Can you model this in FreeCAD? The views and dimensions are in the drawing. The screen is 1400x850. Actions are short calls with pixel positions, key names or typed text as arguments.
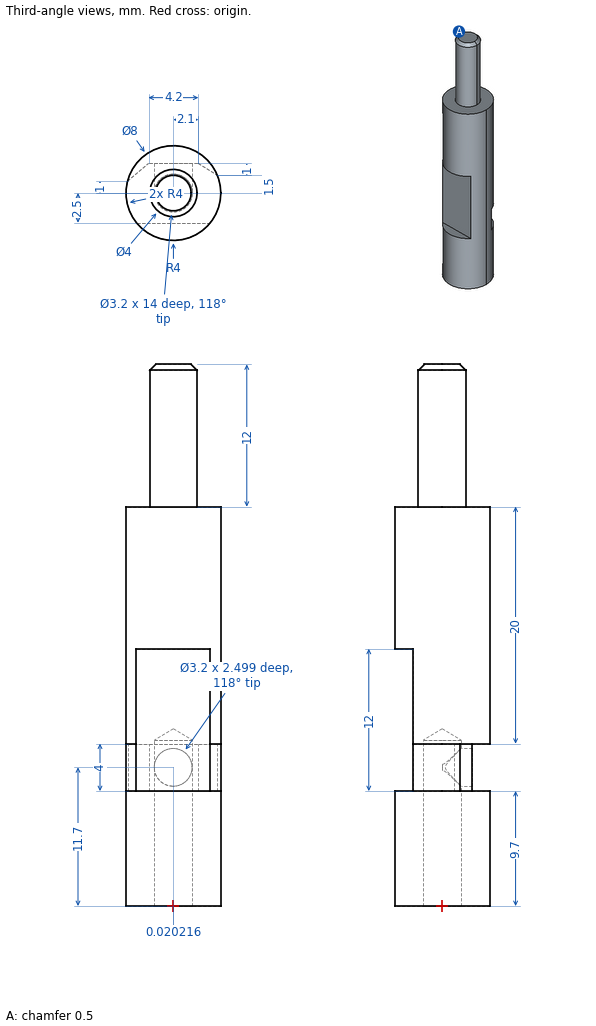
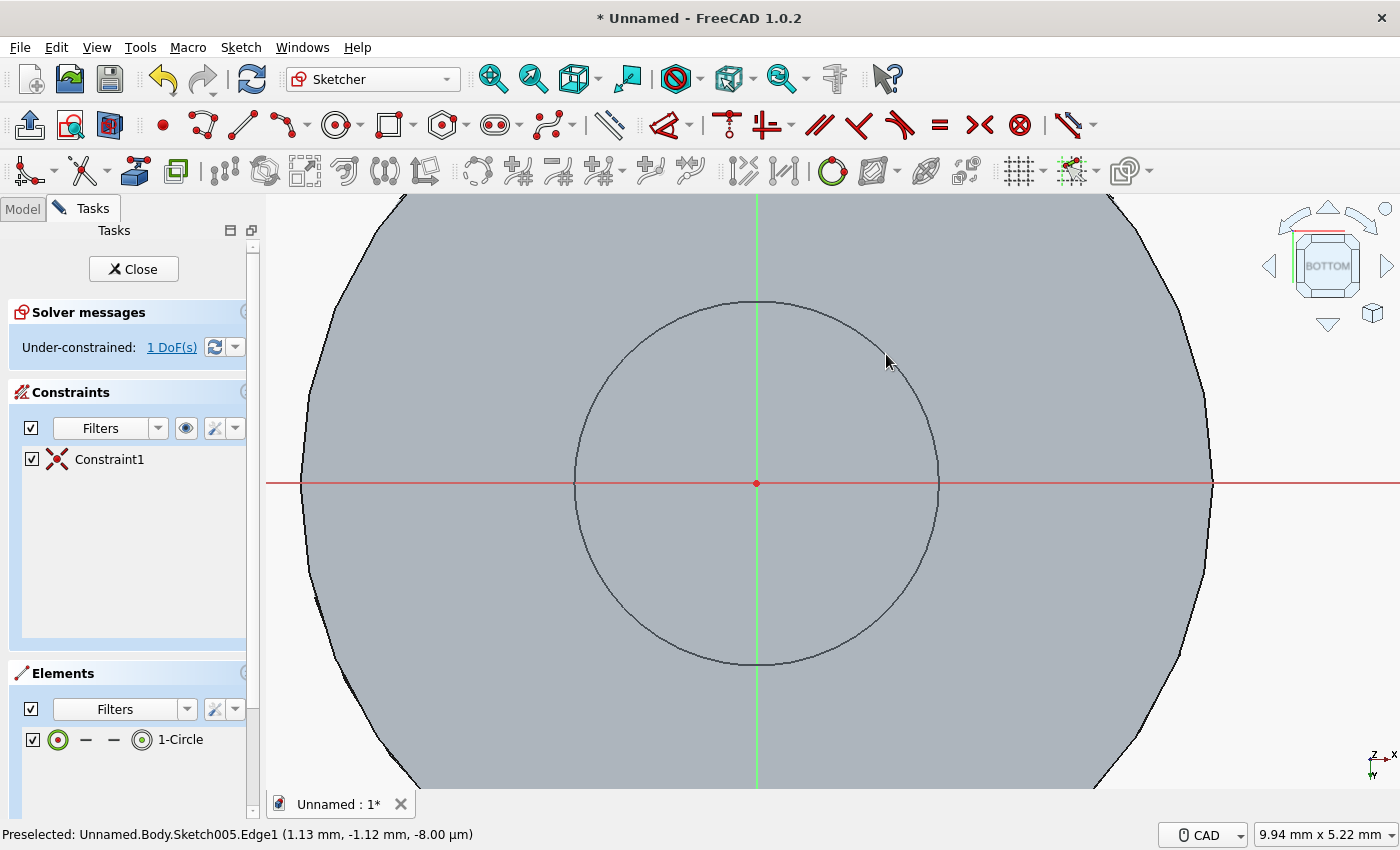
click(664, 126)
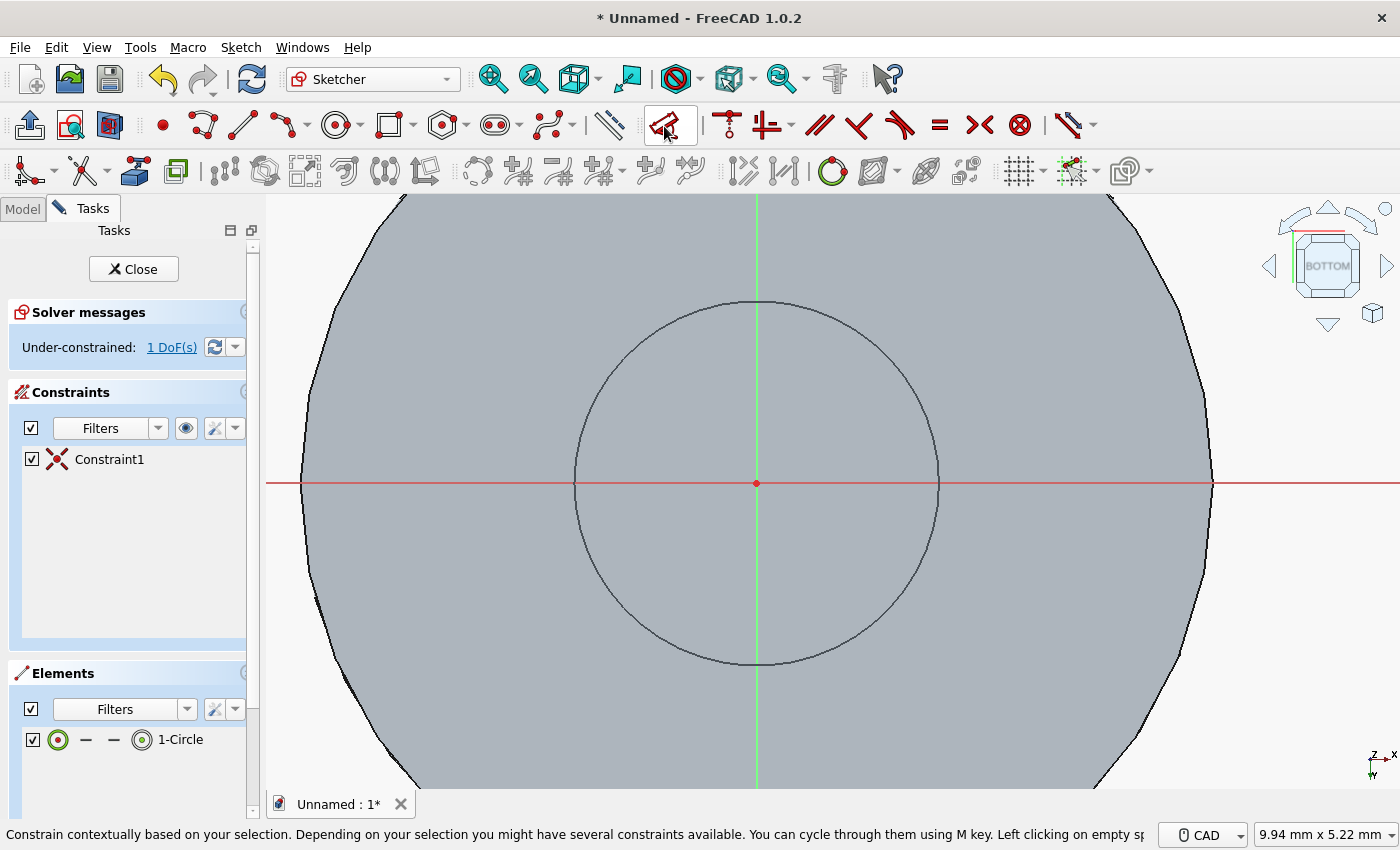
click(885, 354)
click(908, 331)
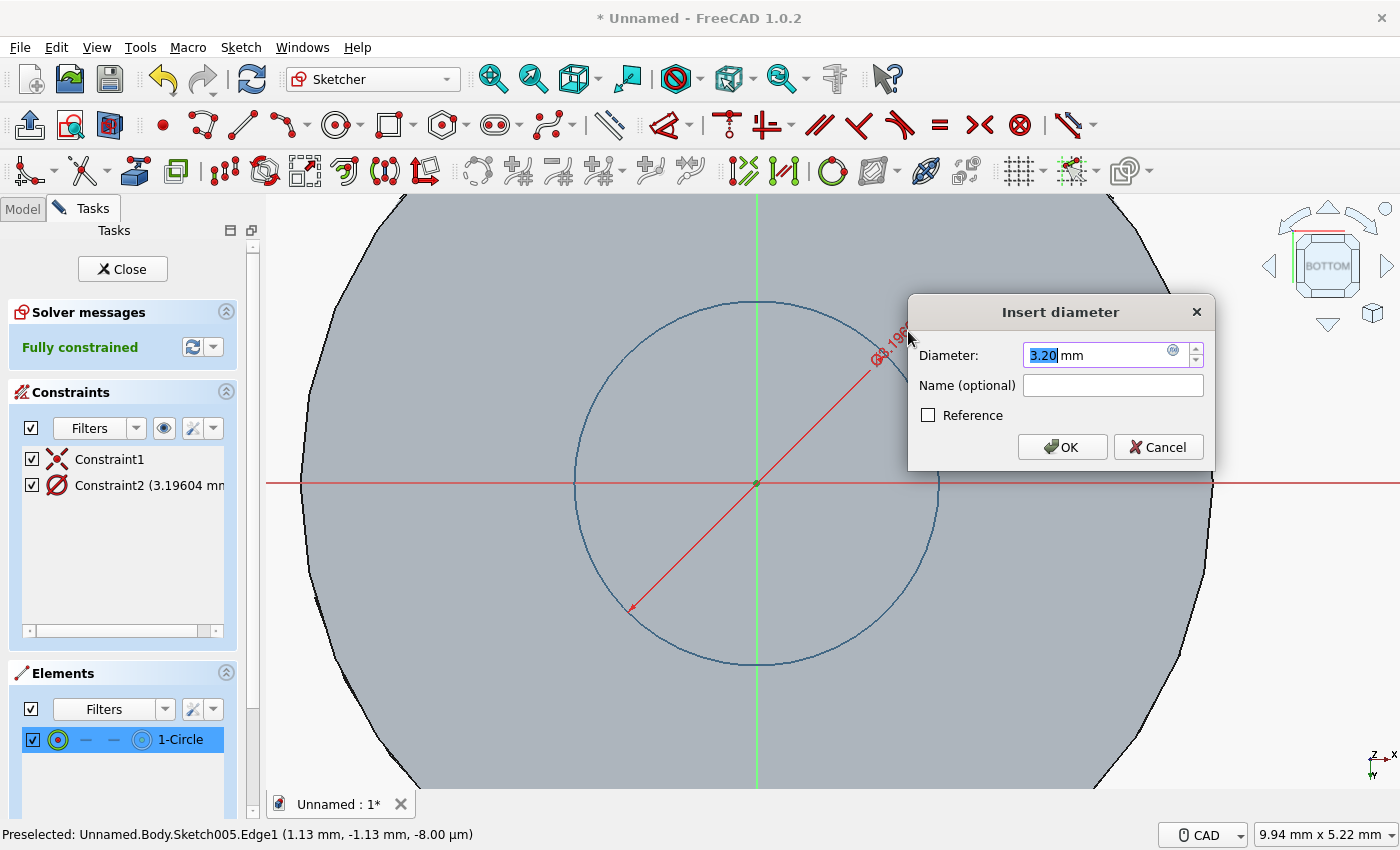
text(3.2)
key(Return)
key(Escape)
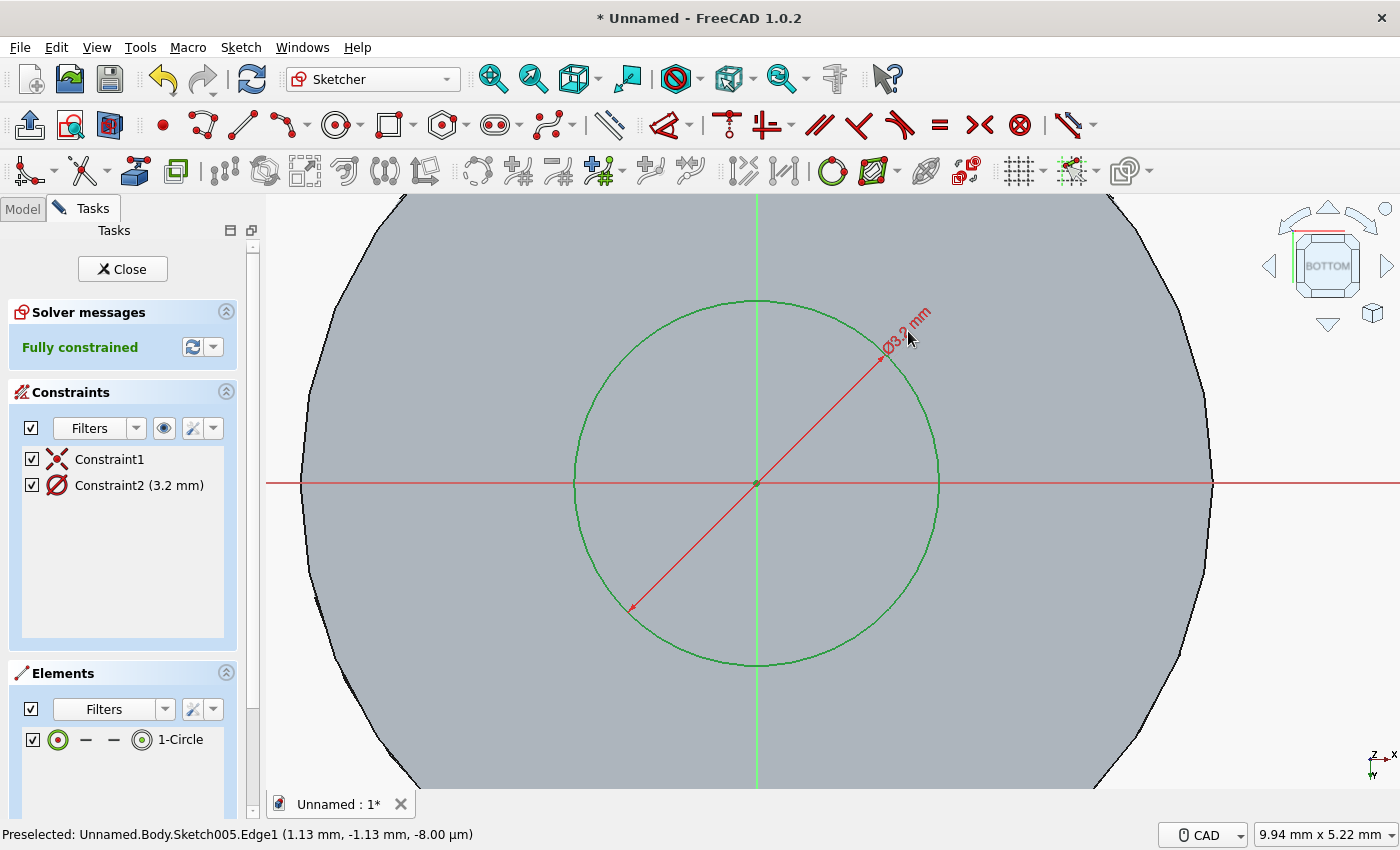
click(123, 269)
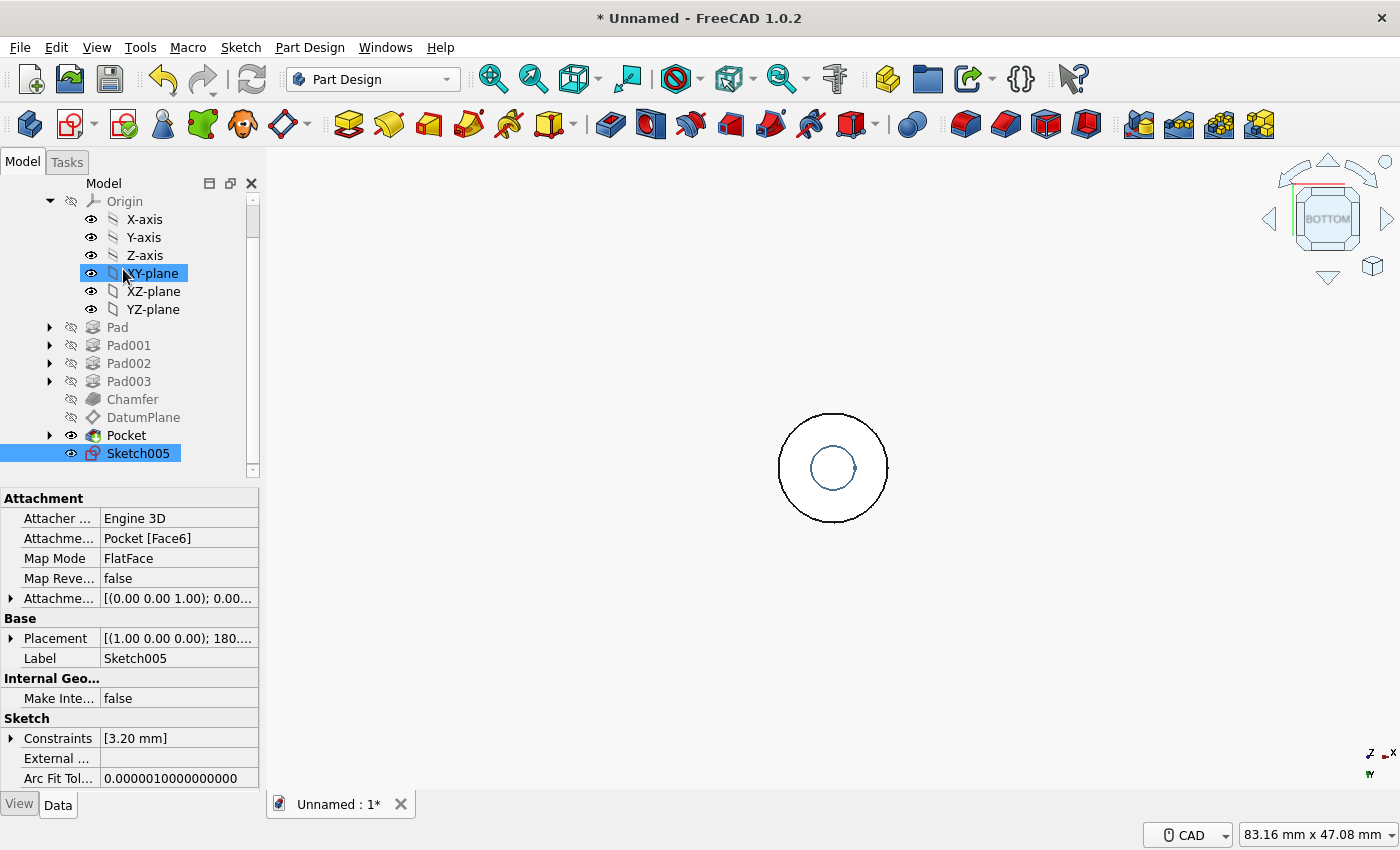
click(652, 124)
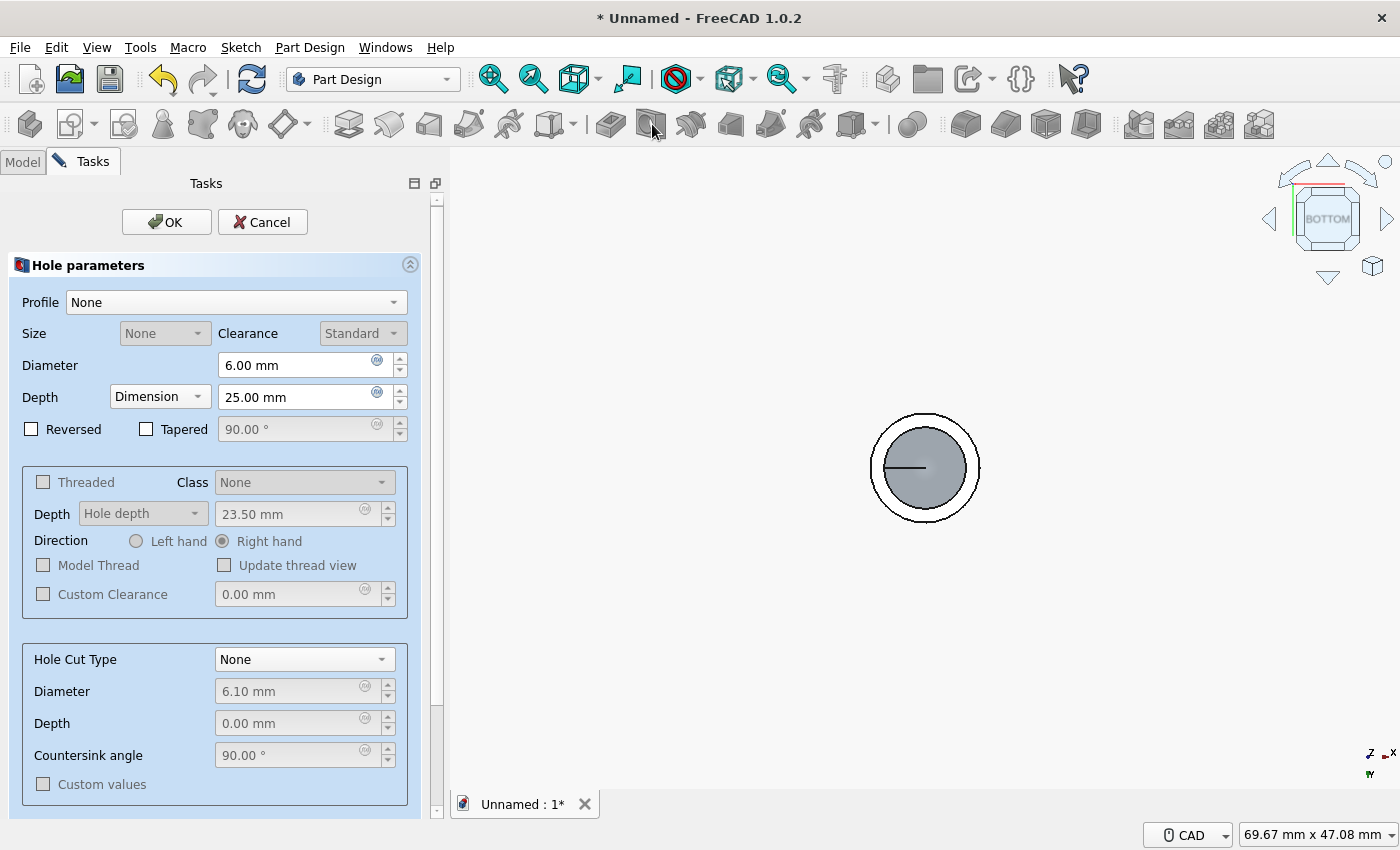
triple_click(305, 365)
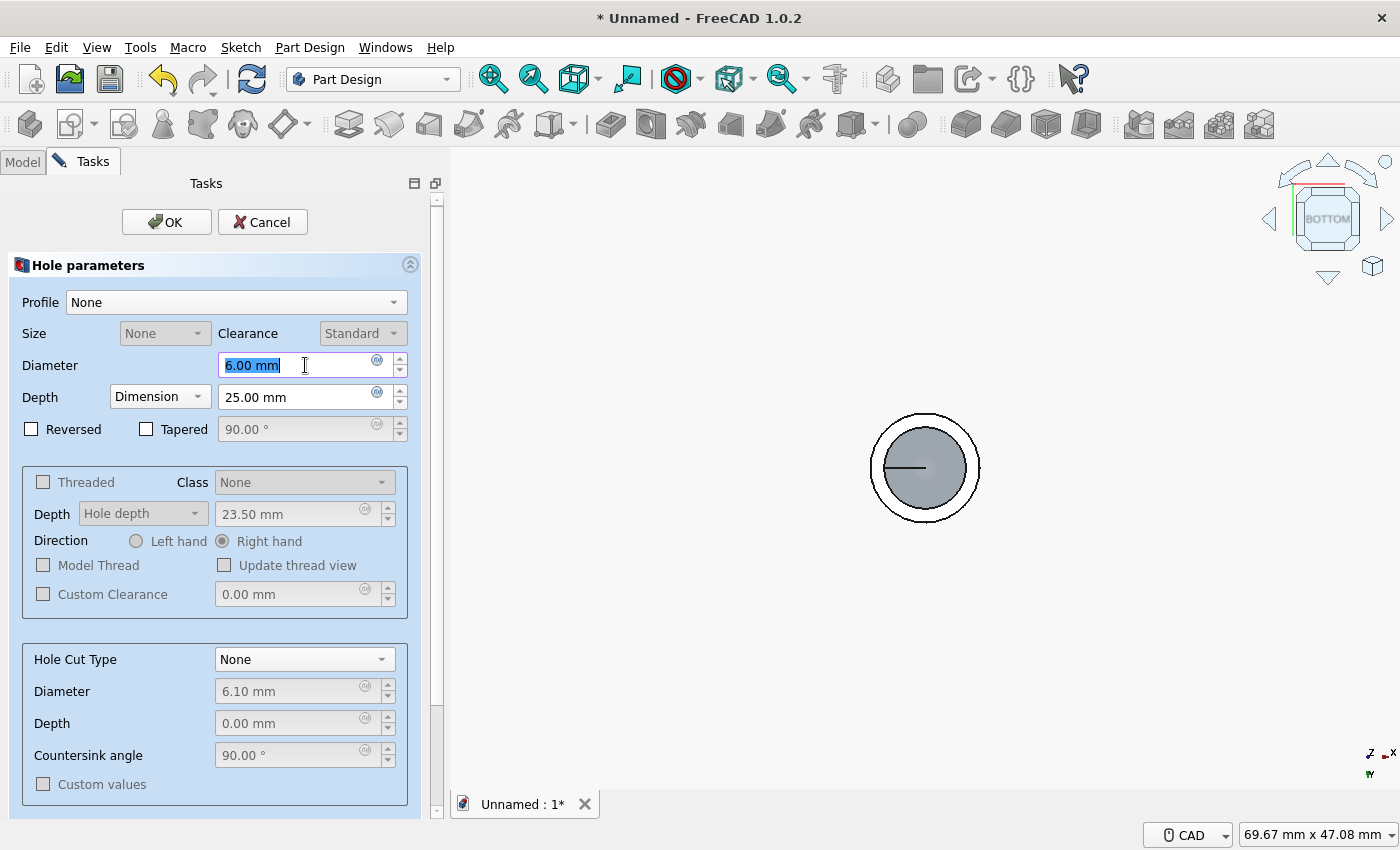
text(3.2)
key(Tab)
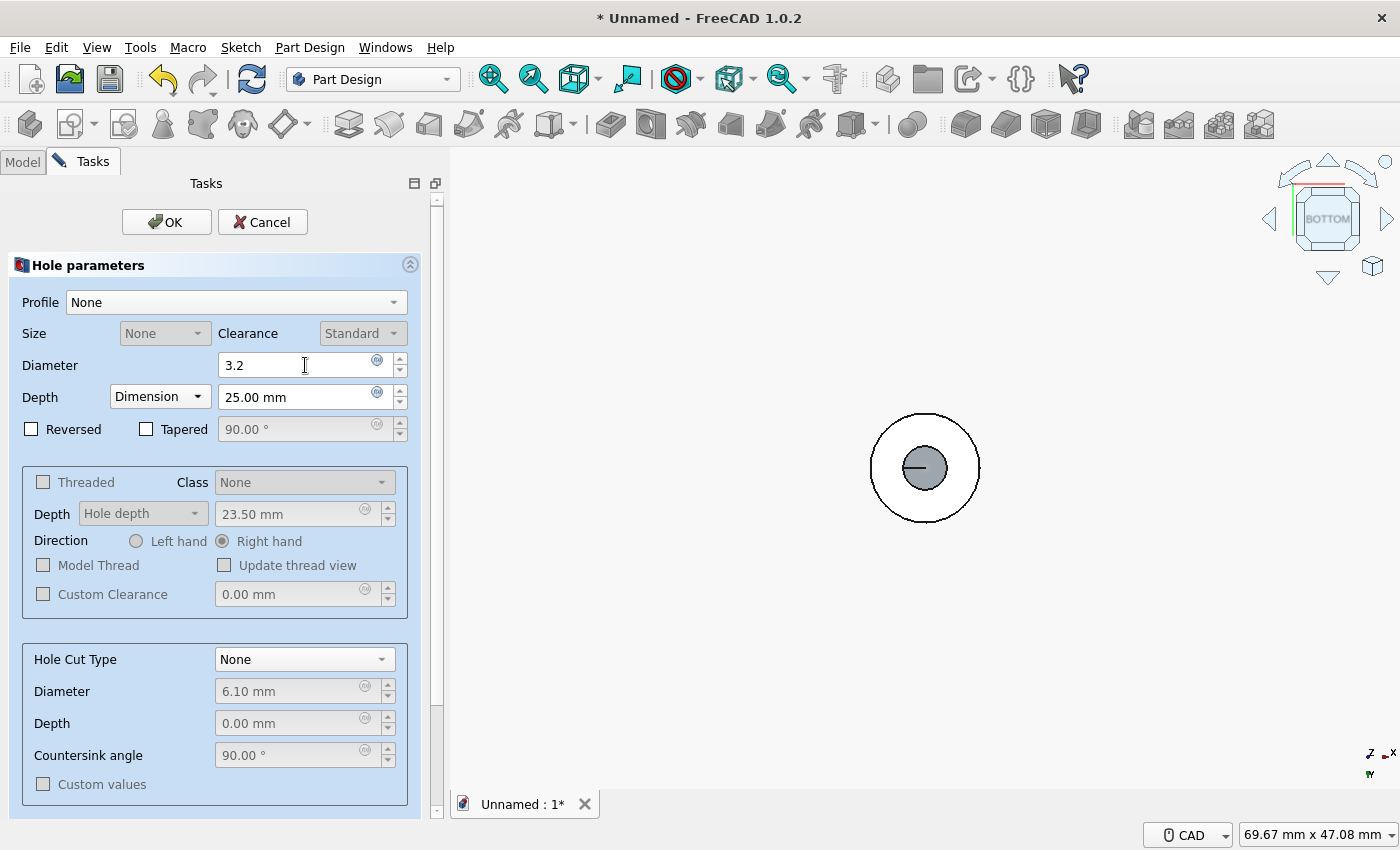
triple_click(305, 397)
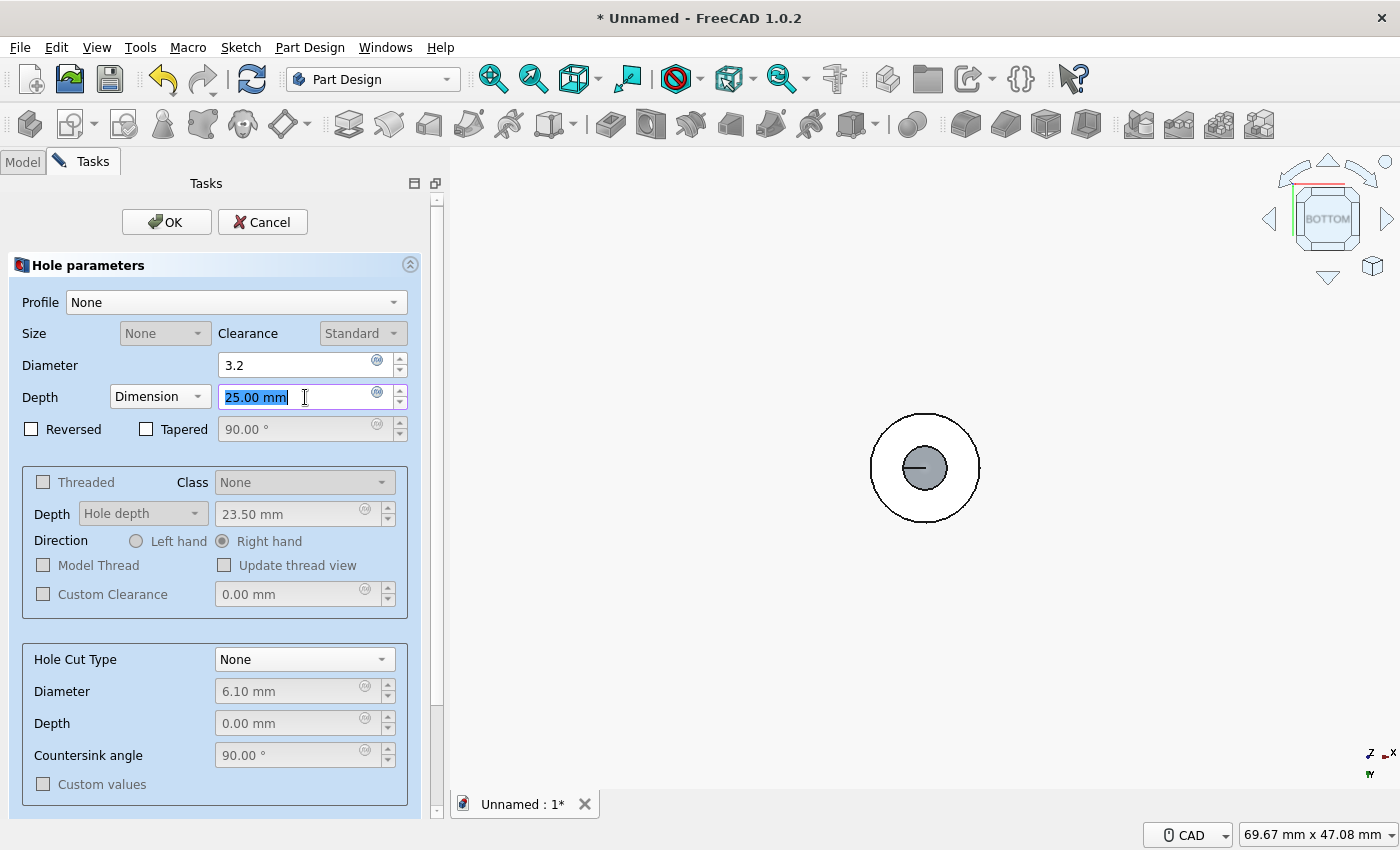
text(14)
key(Tab)